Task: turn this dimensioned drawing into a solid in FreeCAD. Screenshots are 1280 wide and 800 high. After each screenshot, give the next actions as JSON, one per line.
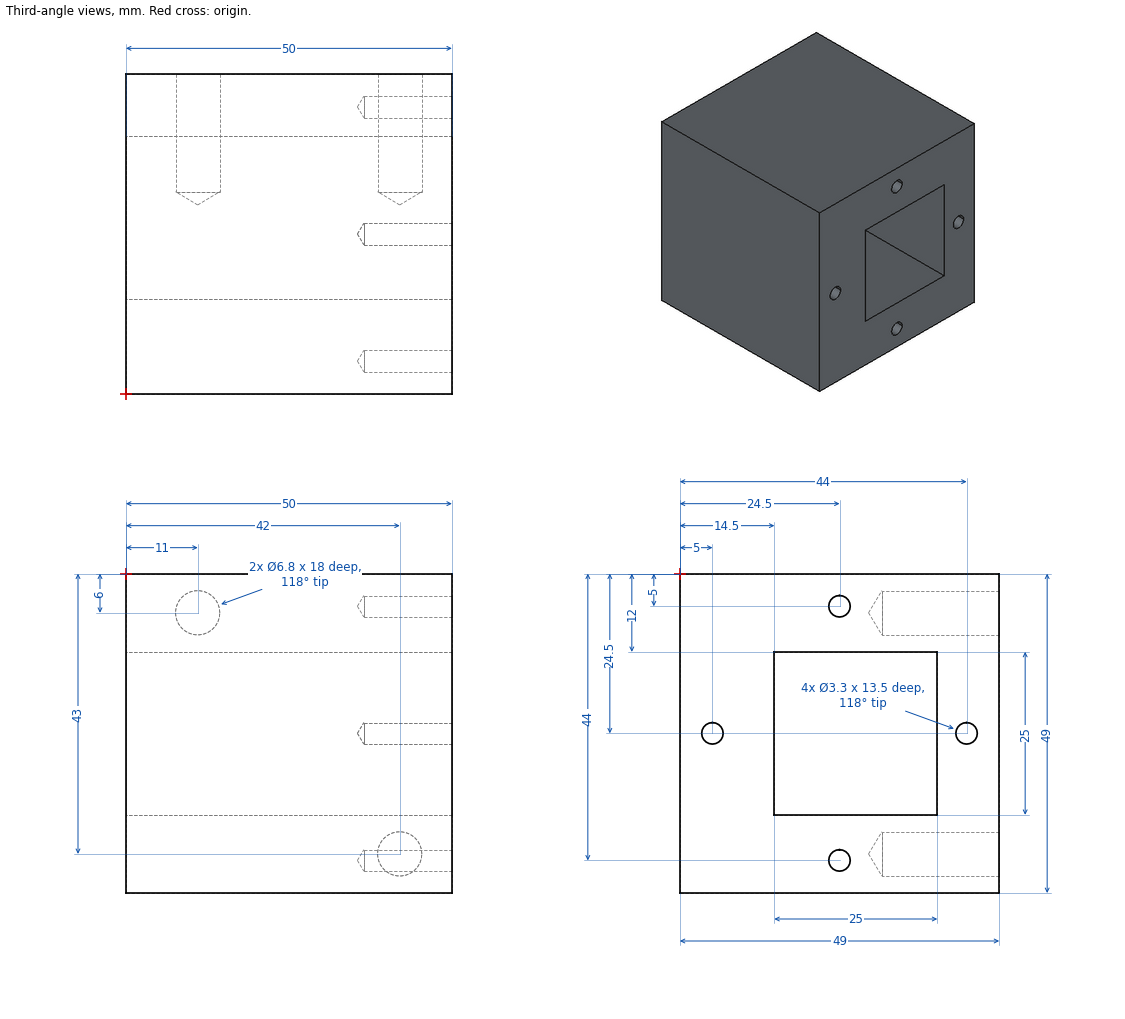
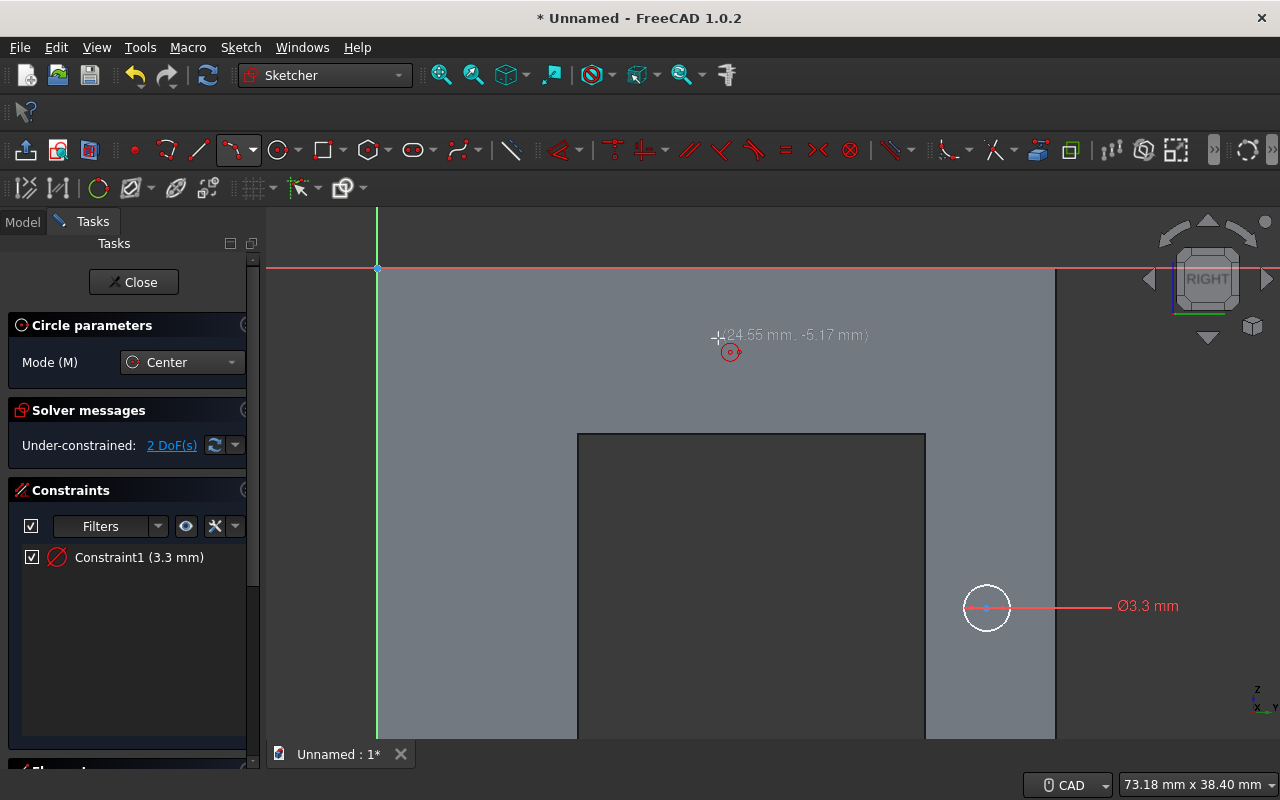
{"action": "left_click", "coordinate": [717, 337]}
{"action": "mouse_move", "coordinate": [733, 321]}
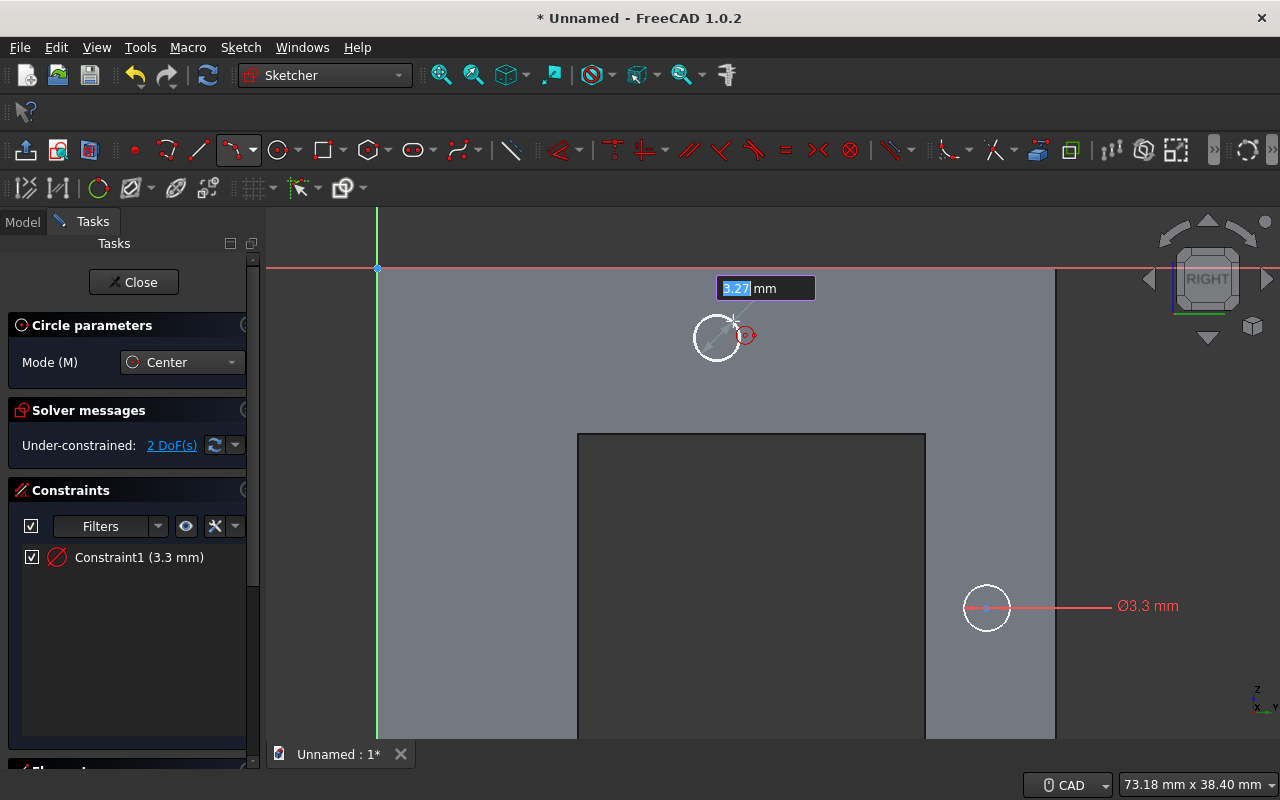
{"action": "type", "text": "3.3"}
{"action": "key", "text": "Return"}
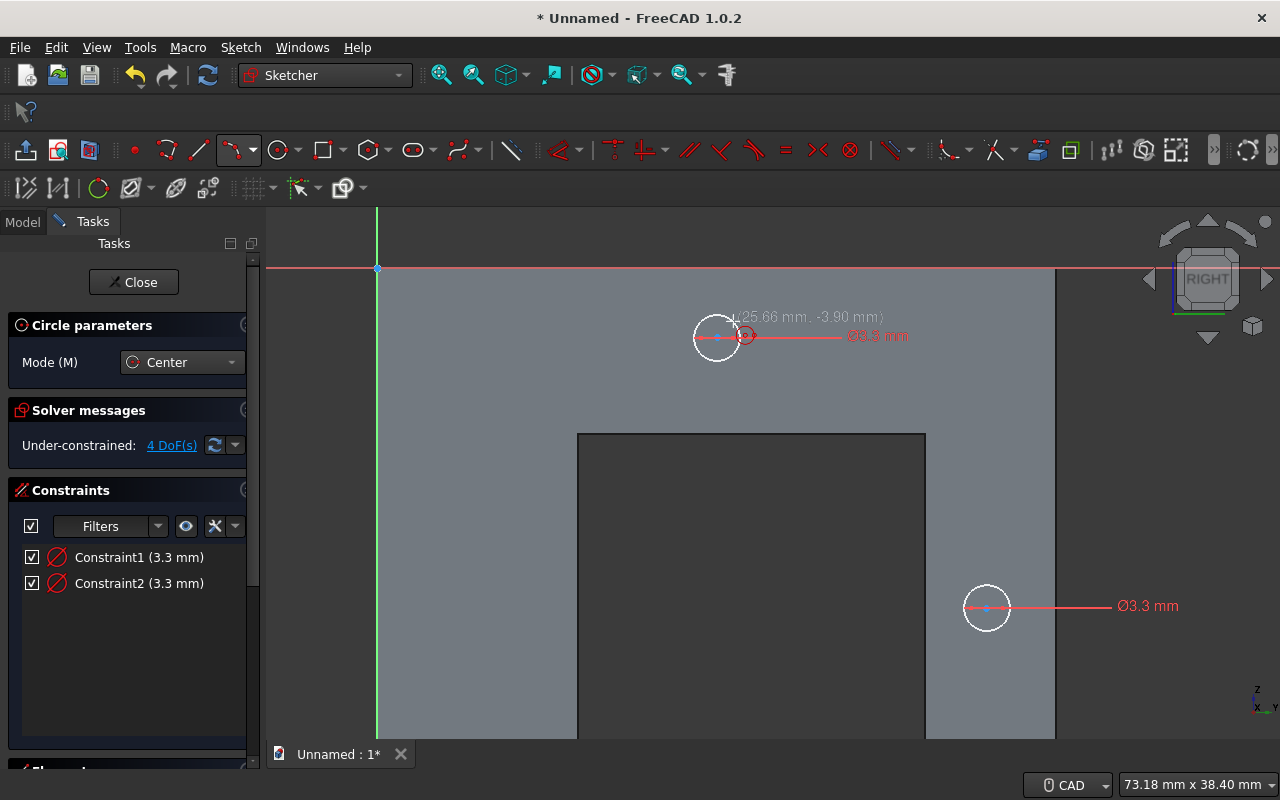
{"action": "left_click", "coordinate": [447, 607]}
{"action": "mouse_move", "coordinate": [463, 591]}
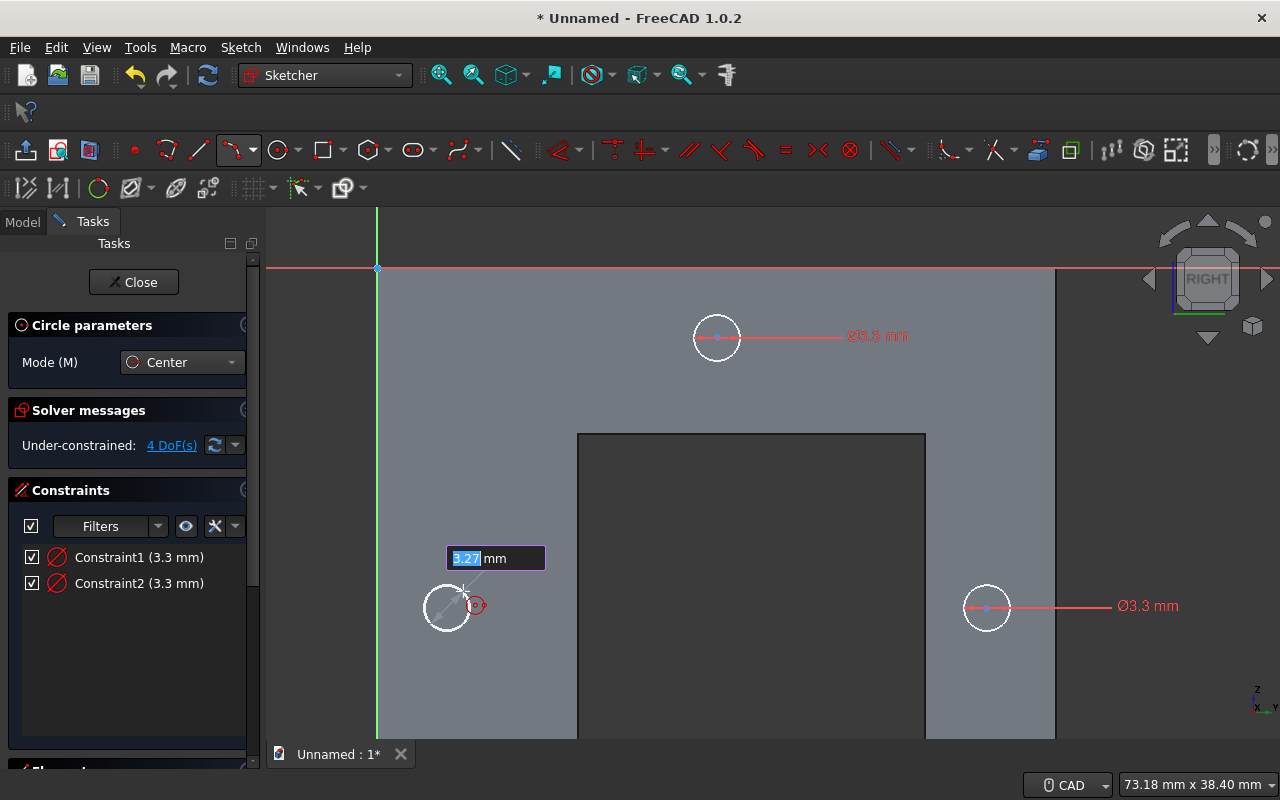
{"action": "type", "text": "3.3"}
{"action": "key", "text": "Return"}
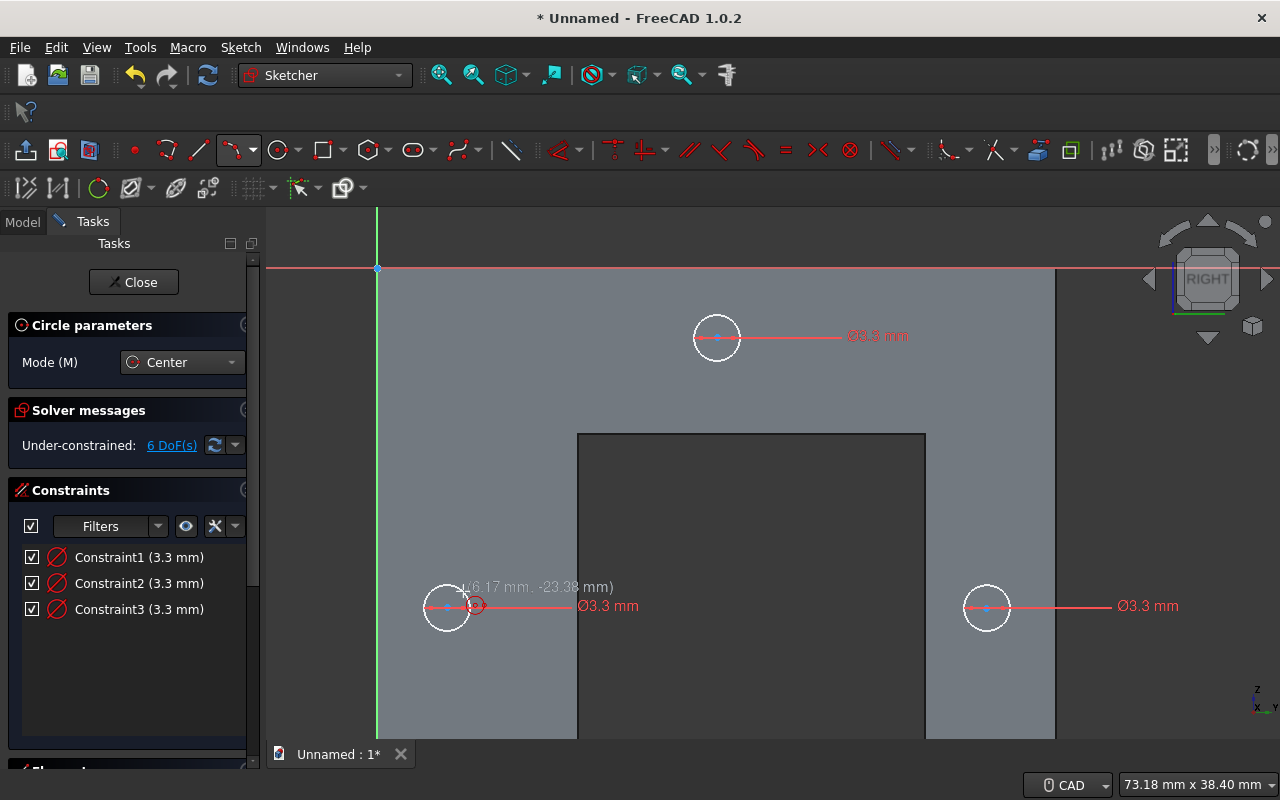
{"action": "scroll", "coordinate": [718, 338], "scroll_direction": "down", "scroll_amount": 3}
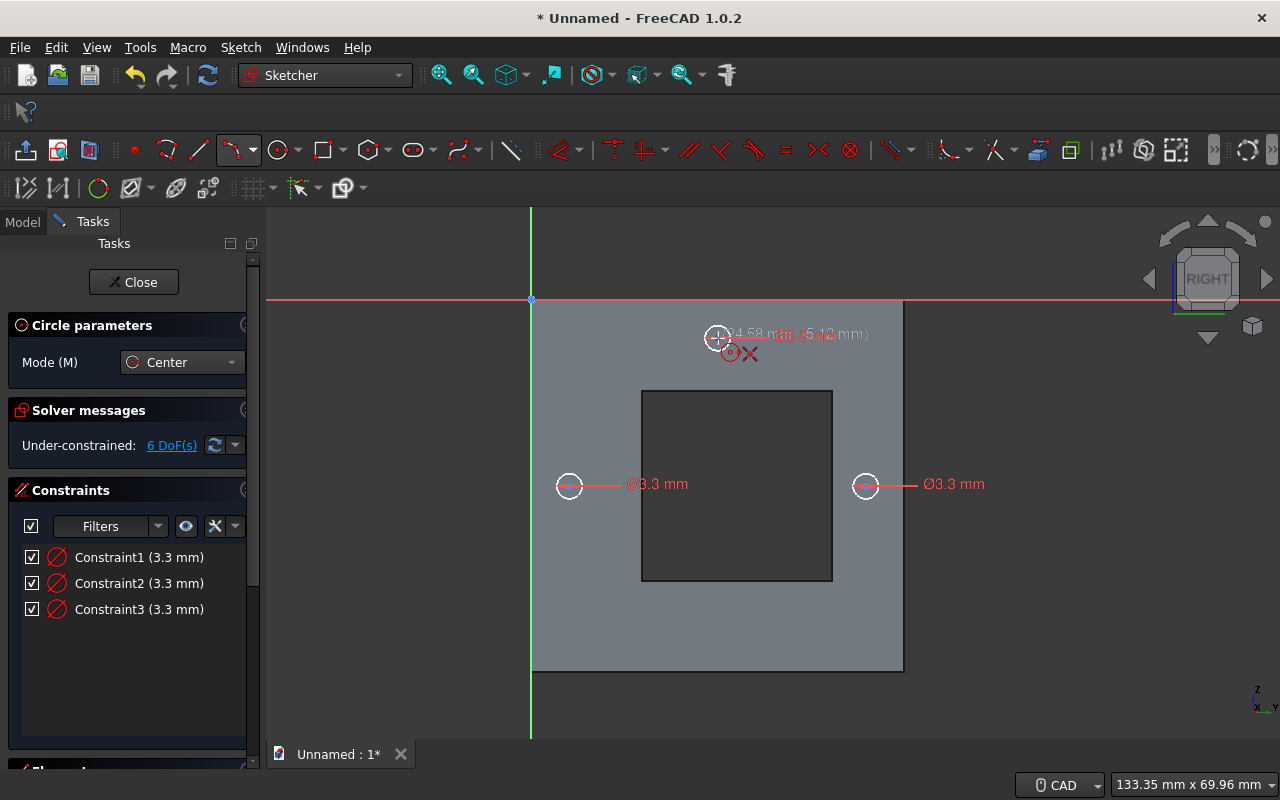
{"action": "scroll", "coordinate": [718, 634], "scroll_direction": "up", "scroll_amount": 3}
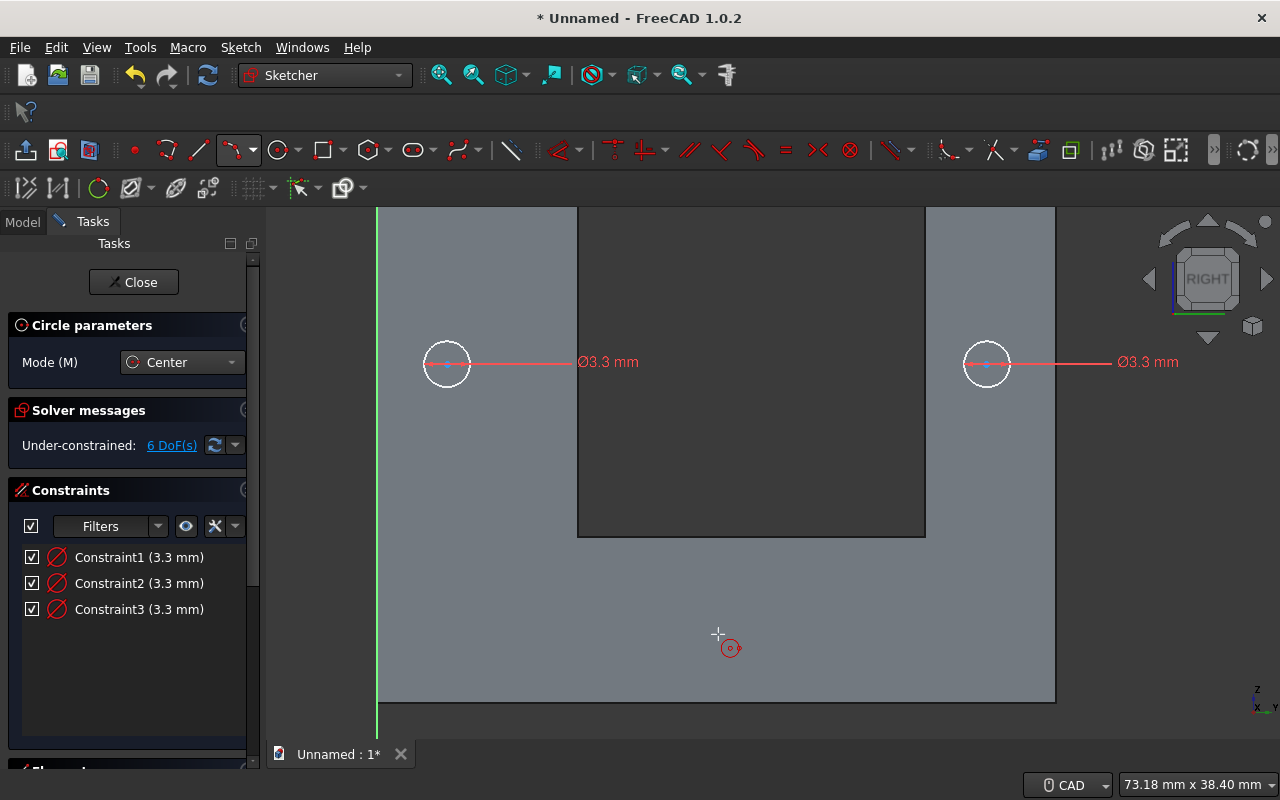
{"action": "left_click", "coordinate": [717, 634]}
{"action": "mouse_move", "coordinate": [733, 618]}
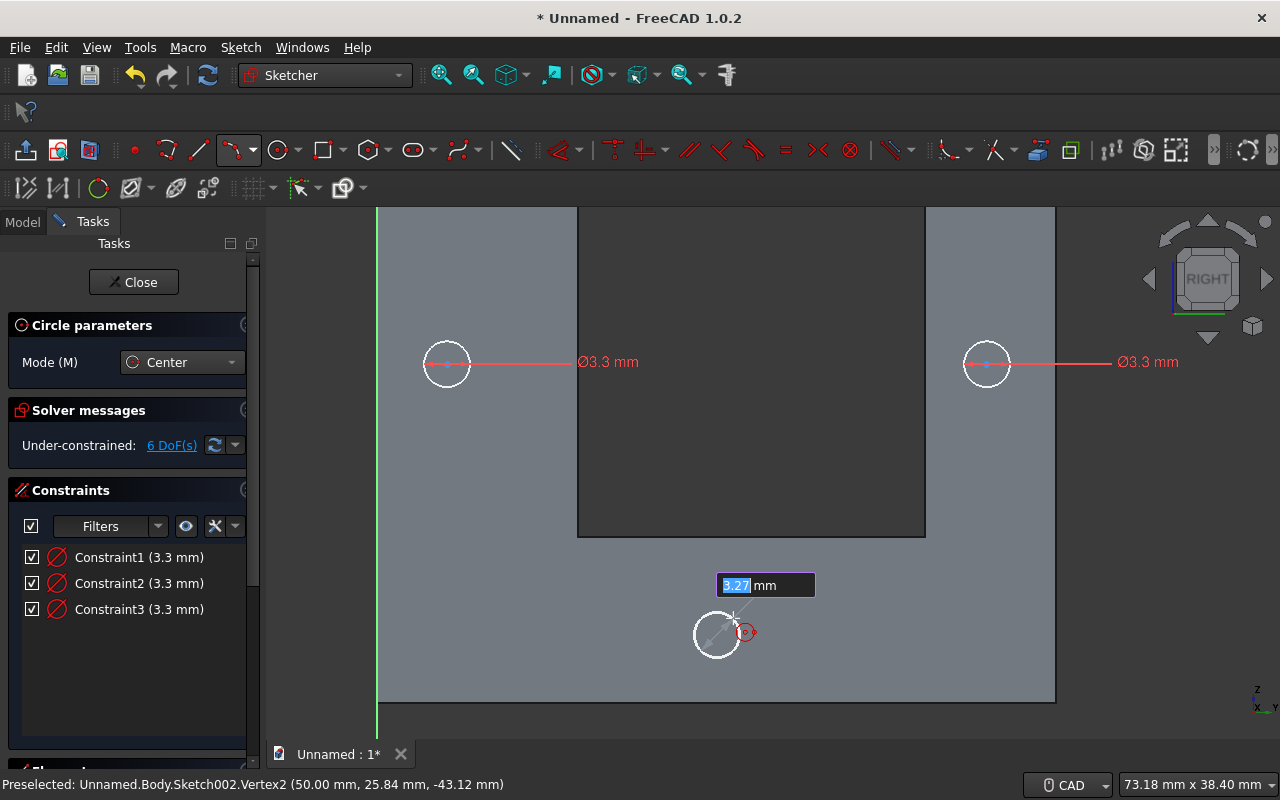
{"action": "type", "text": "3.3"}
{"action": "key", "text": "Return"}
{"action": "key", "text": "Escape"}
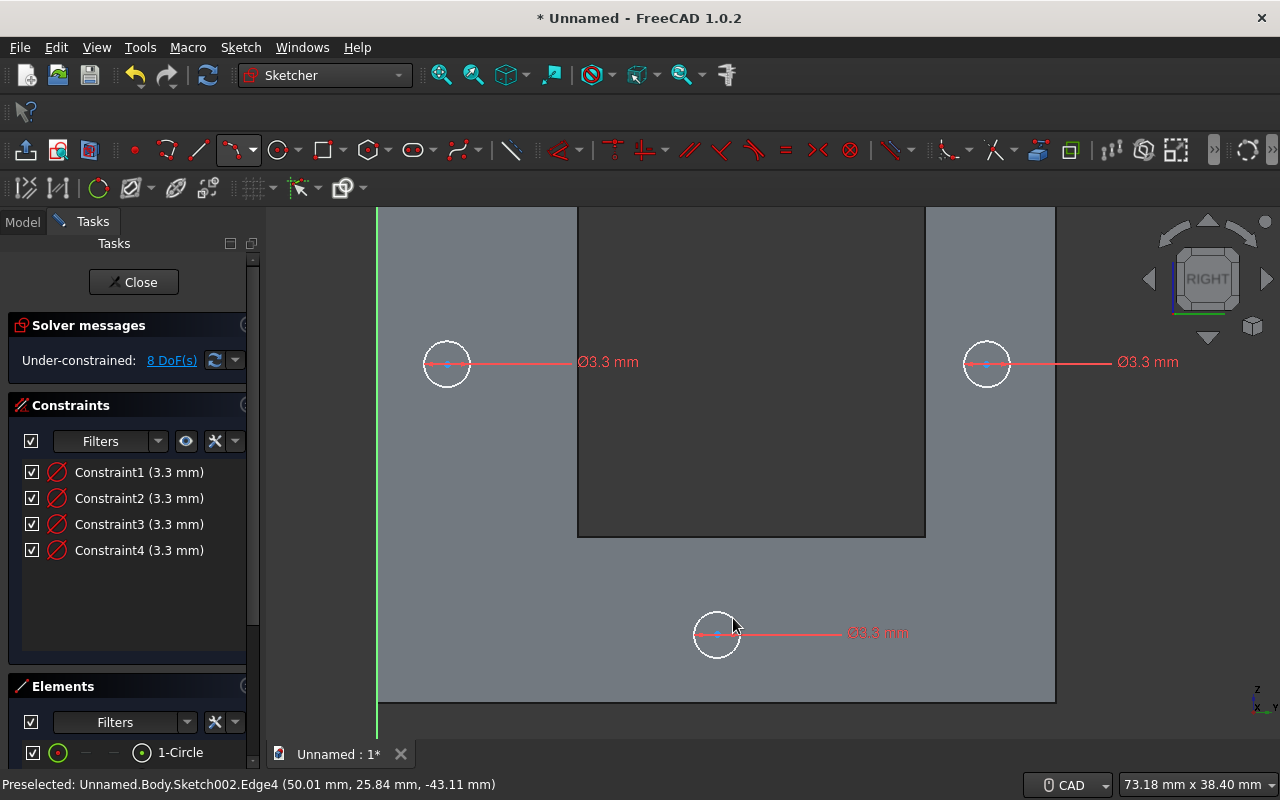
{"action": "left_click", "coordinate": [987, 364]}